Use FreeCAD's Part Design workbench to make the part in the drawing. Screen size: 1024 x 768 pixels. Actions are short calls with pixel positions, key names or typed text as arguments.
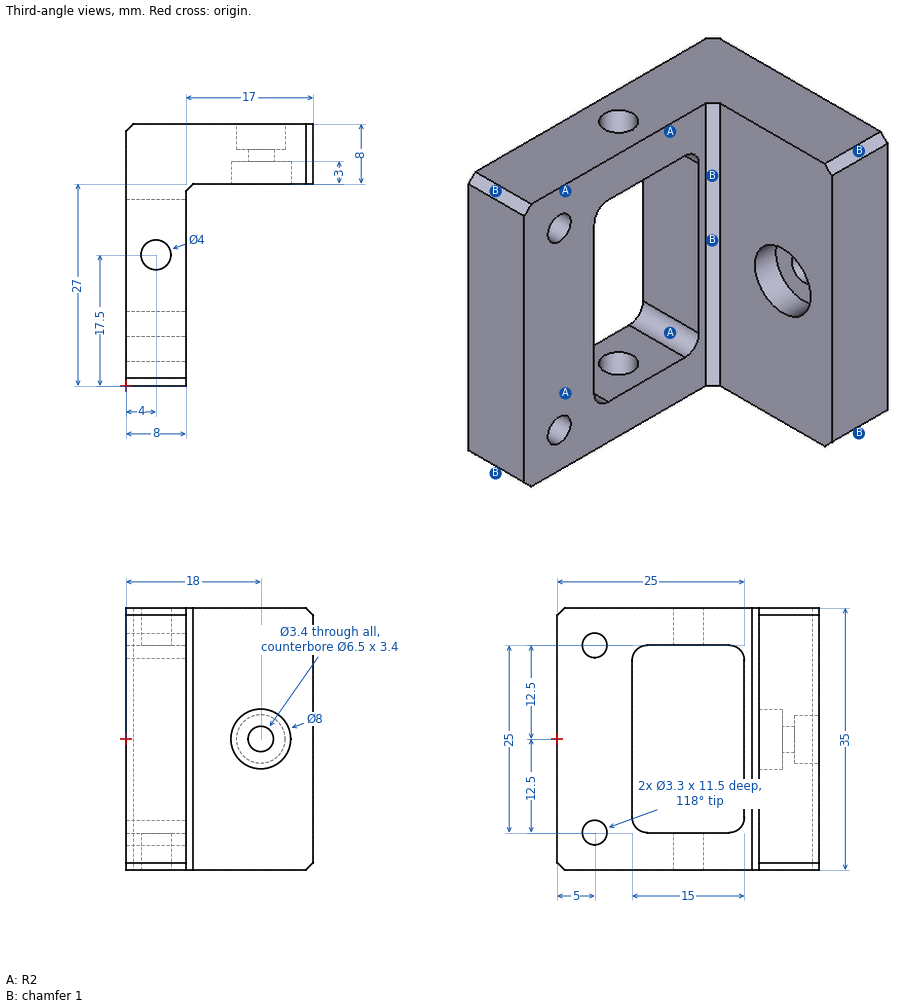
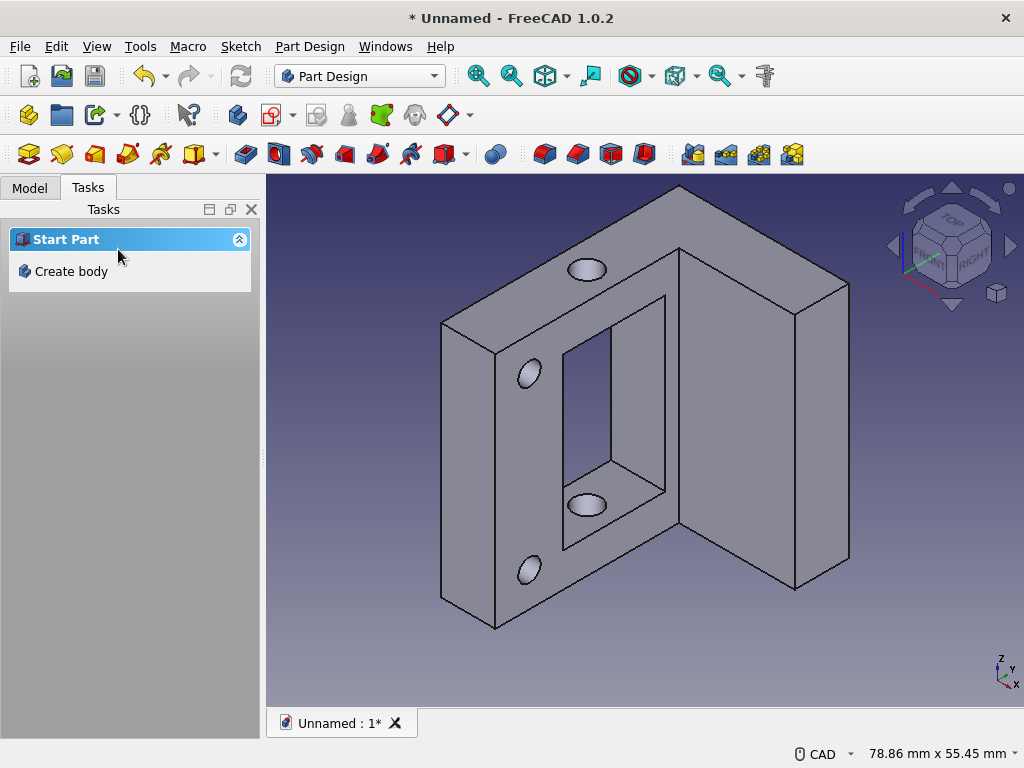
key(1)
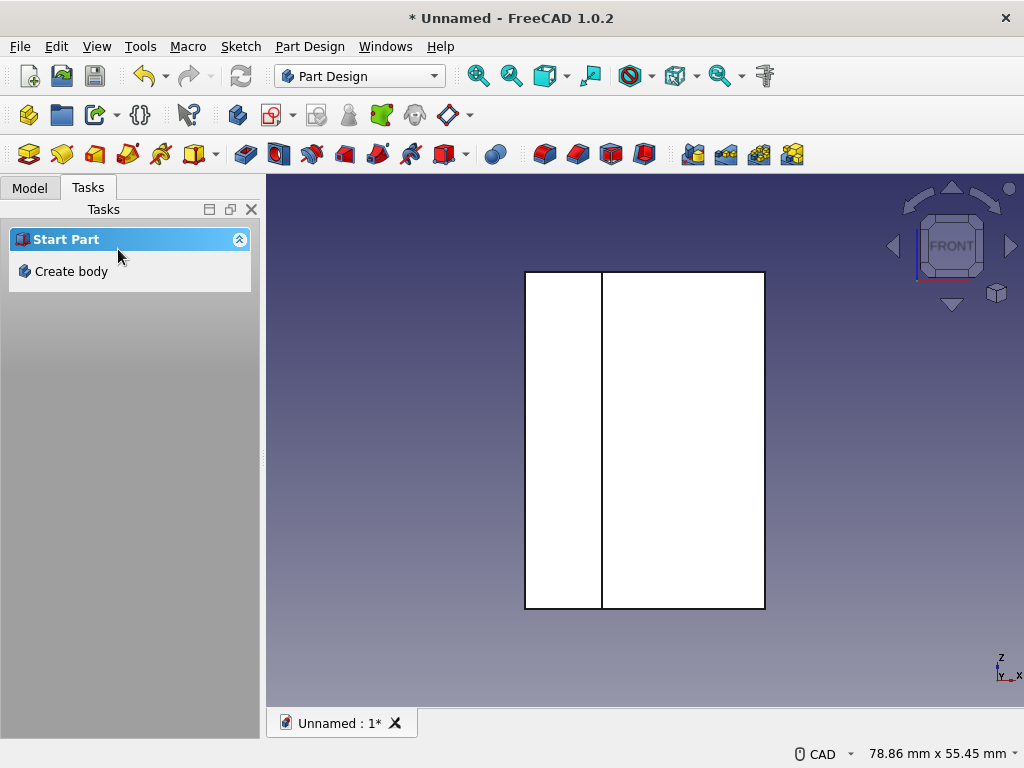
key(3)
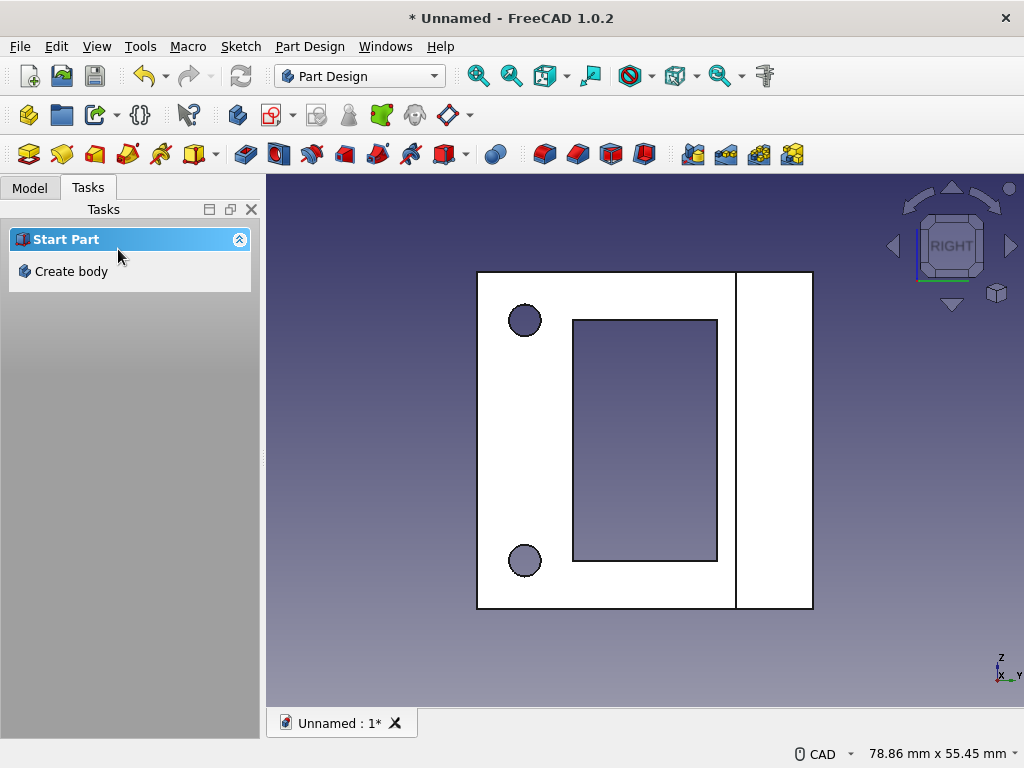
key(5)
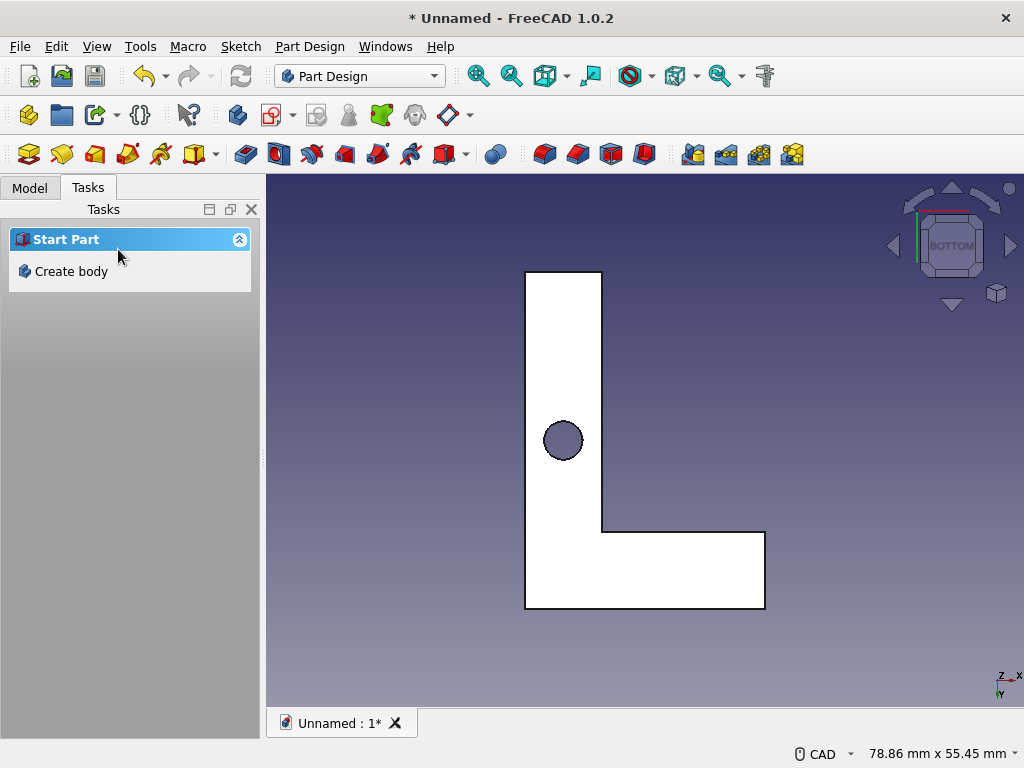
key(4)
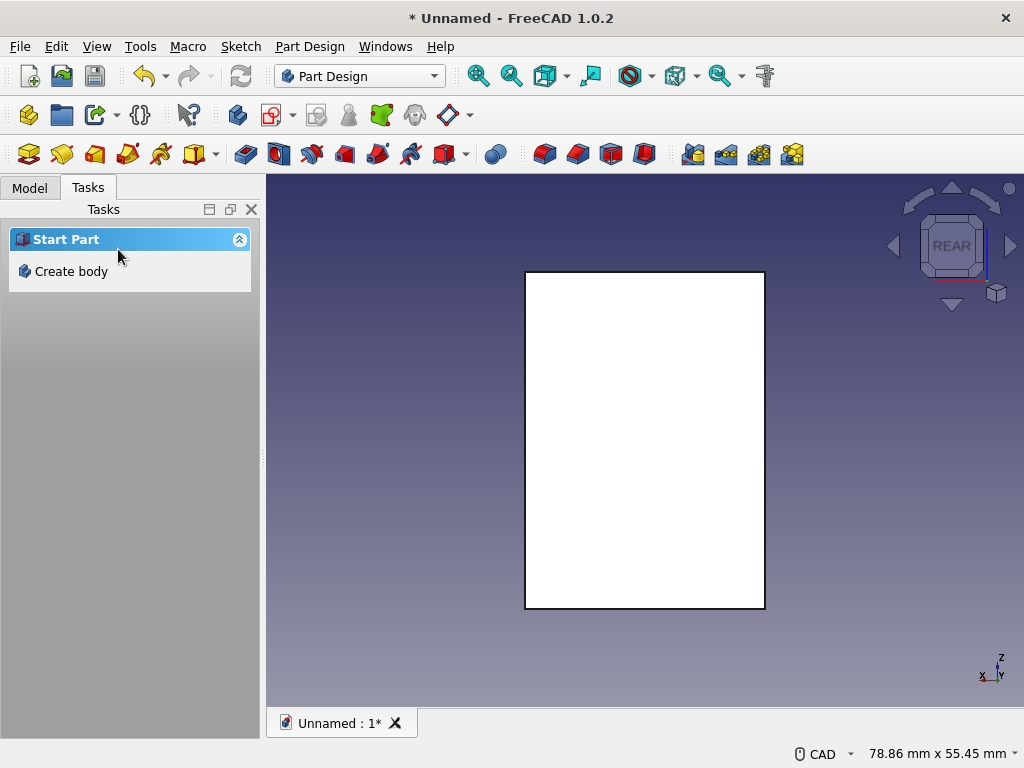
key(6)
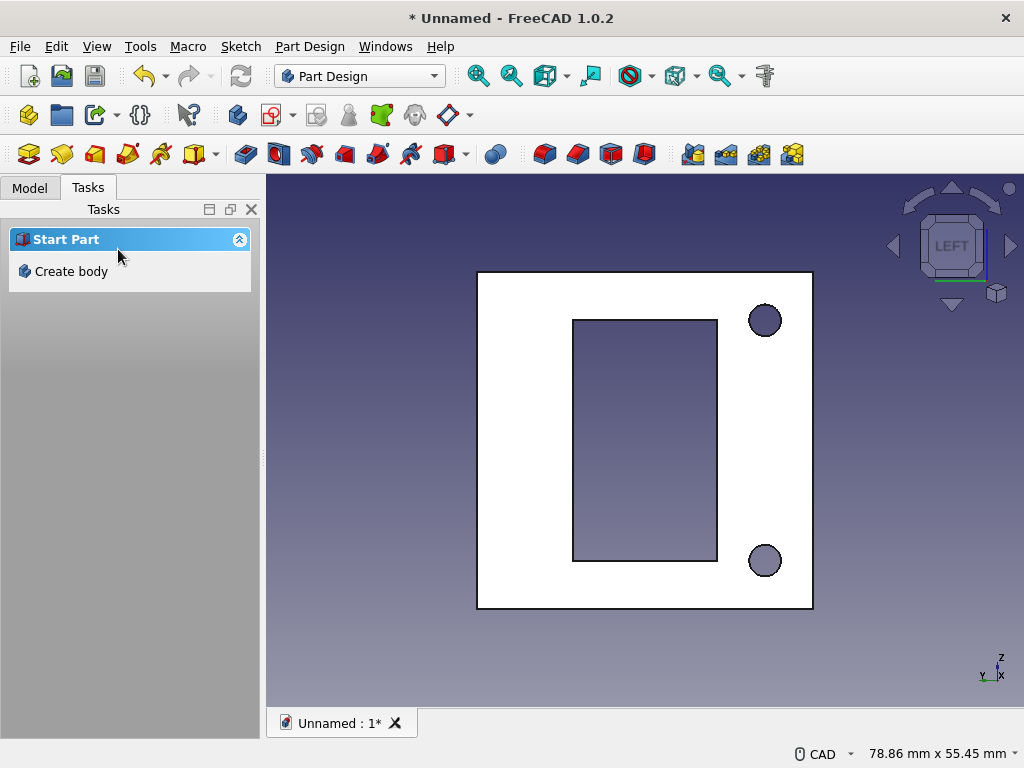
key(v)
key(3)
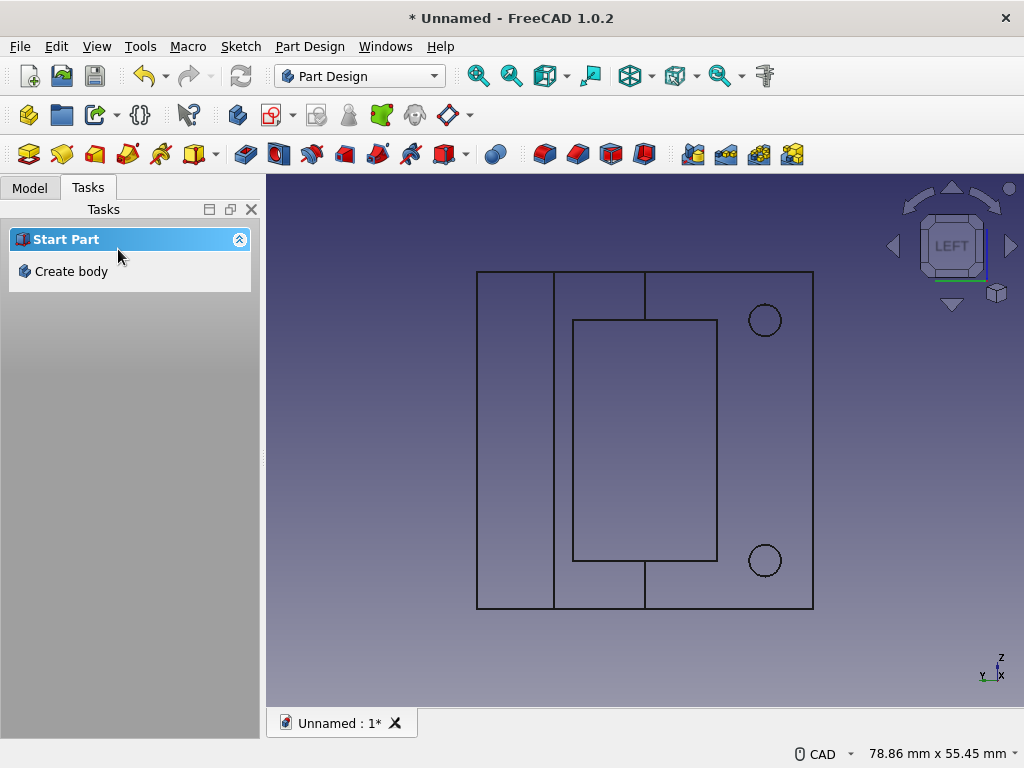
key(0)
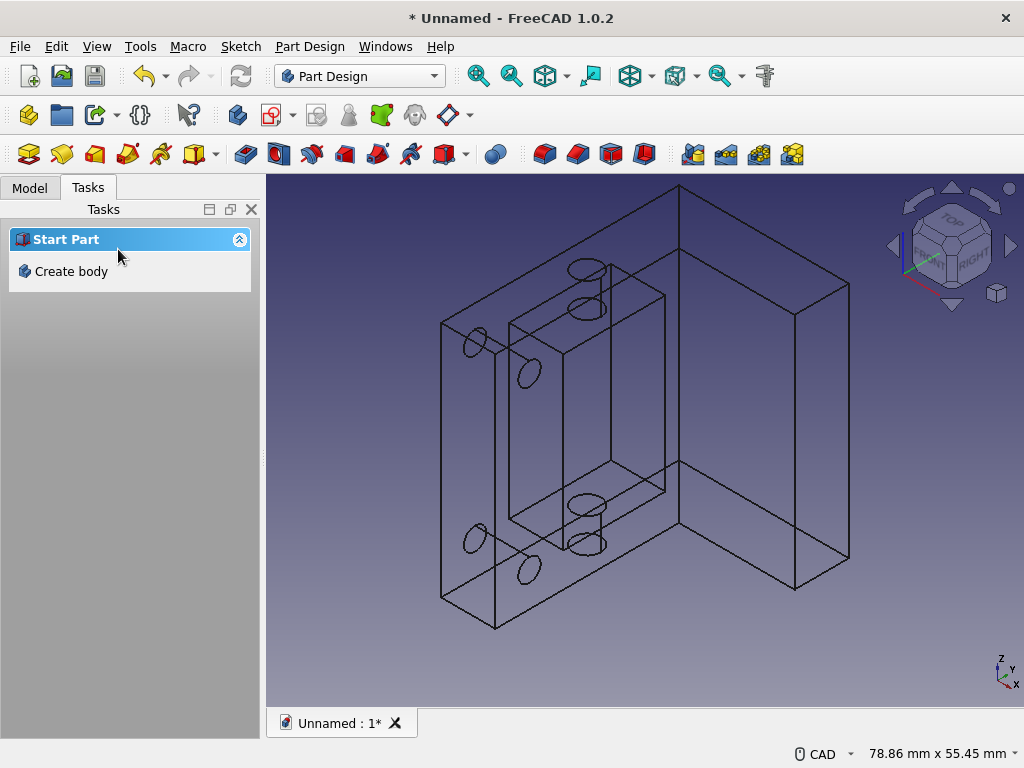
click(536, 534)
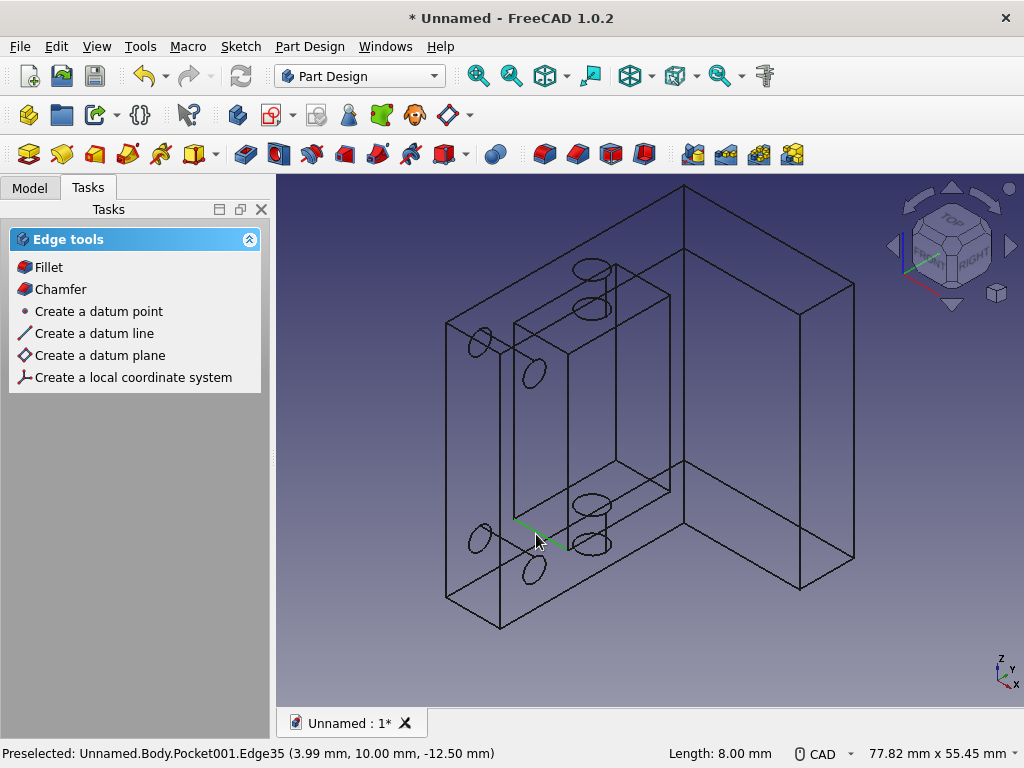
click(643, 475, ctrl)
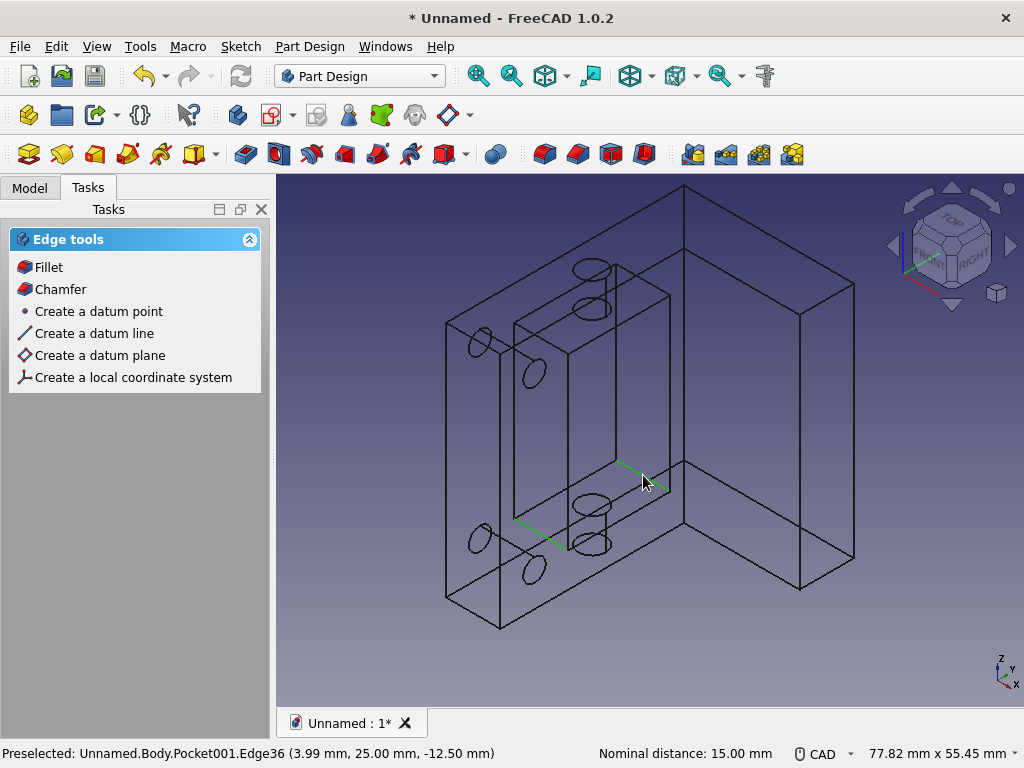
click(643, 279, ctrl)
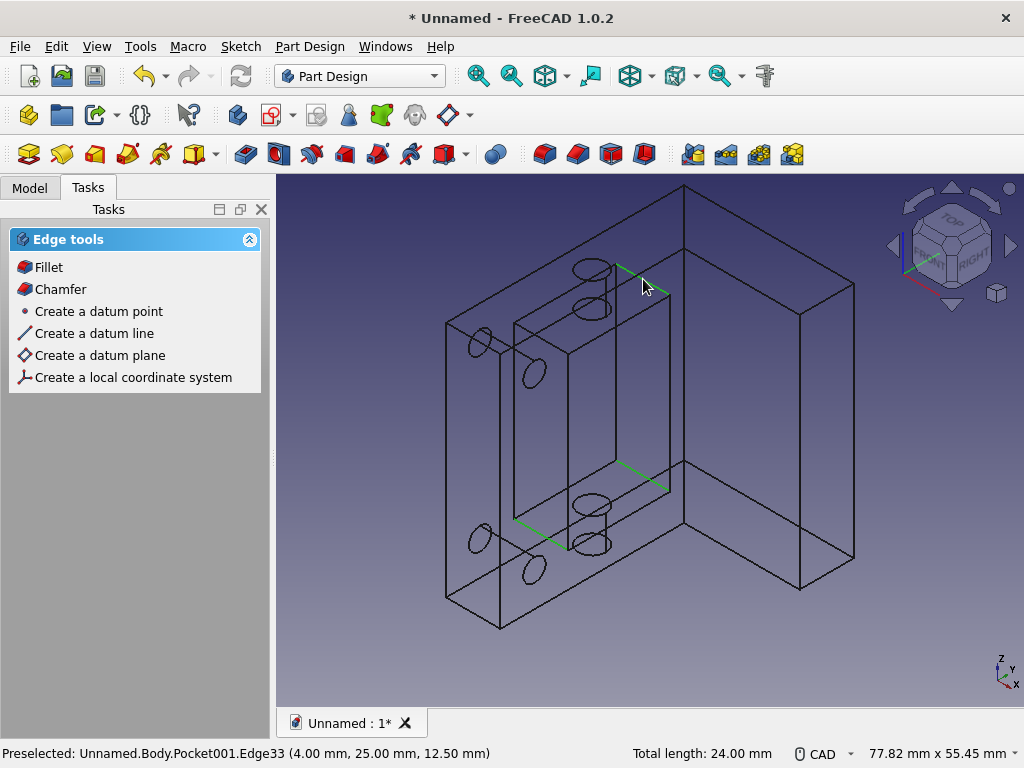
click(547, 341, ctrl)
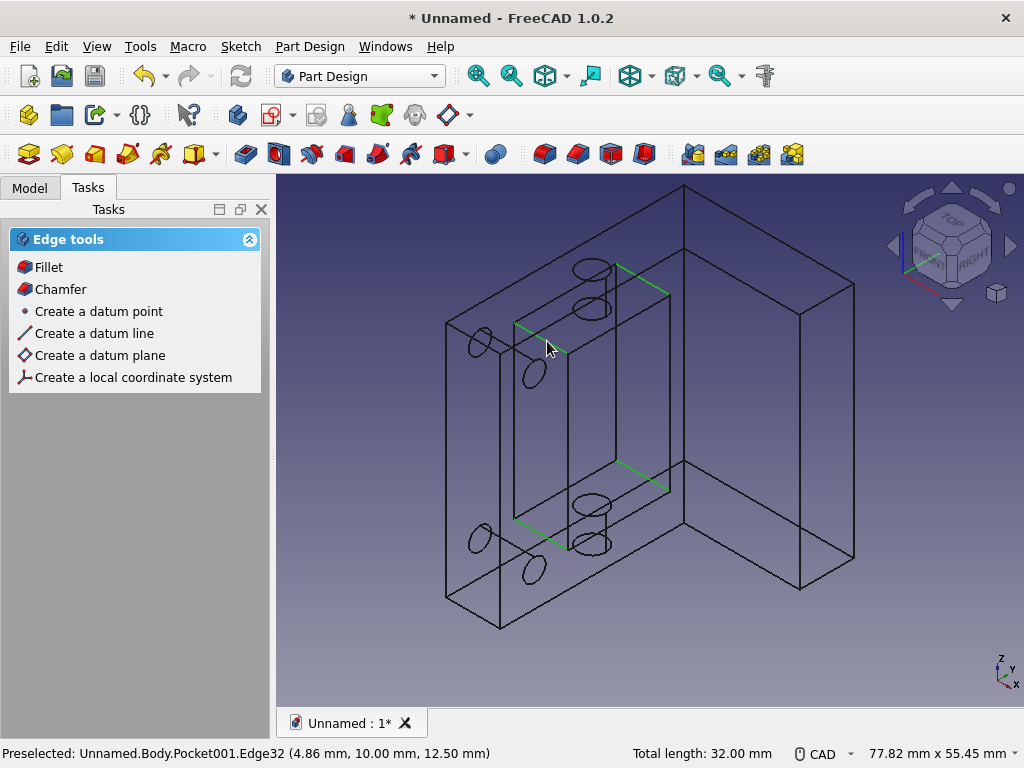
key(v)
key(1)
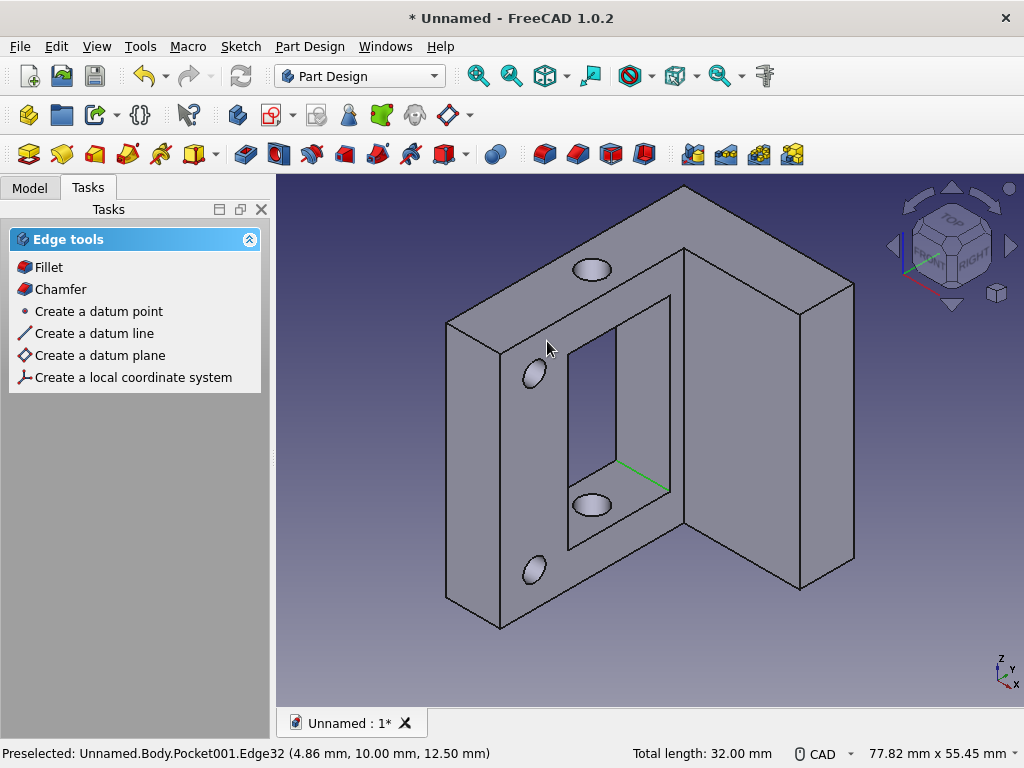
click(545, 154)